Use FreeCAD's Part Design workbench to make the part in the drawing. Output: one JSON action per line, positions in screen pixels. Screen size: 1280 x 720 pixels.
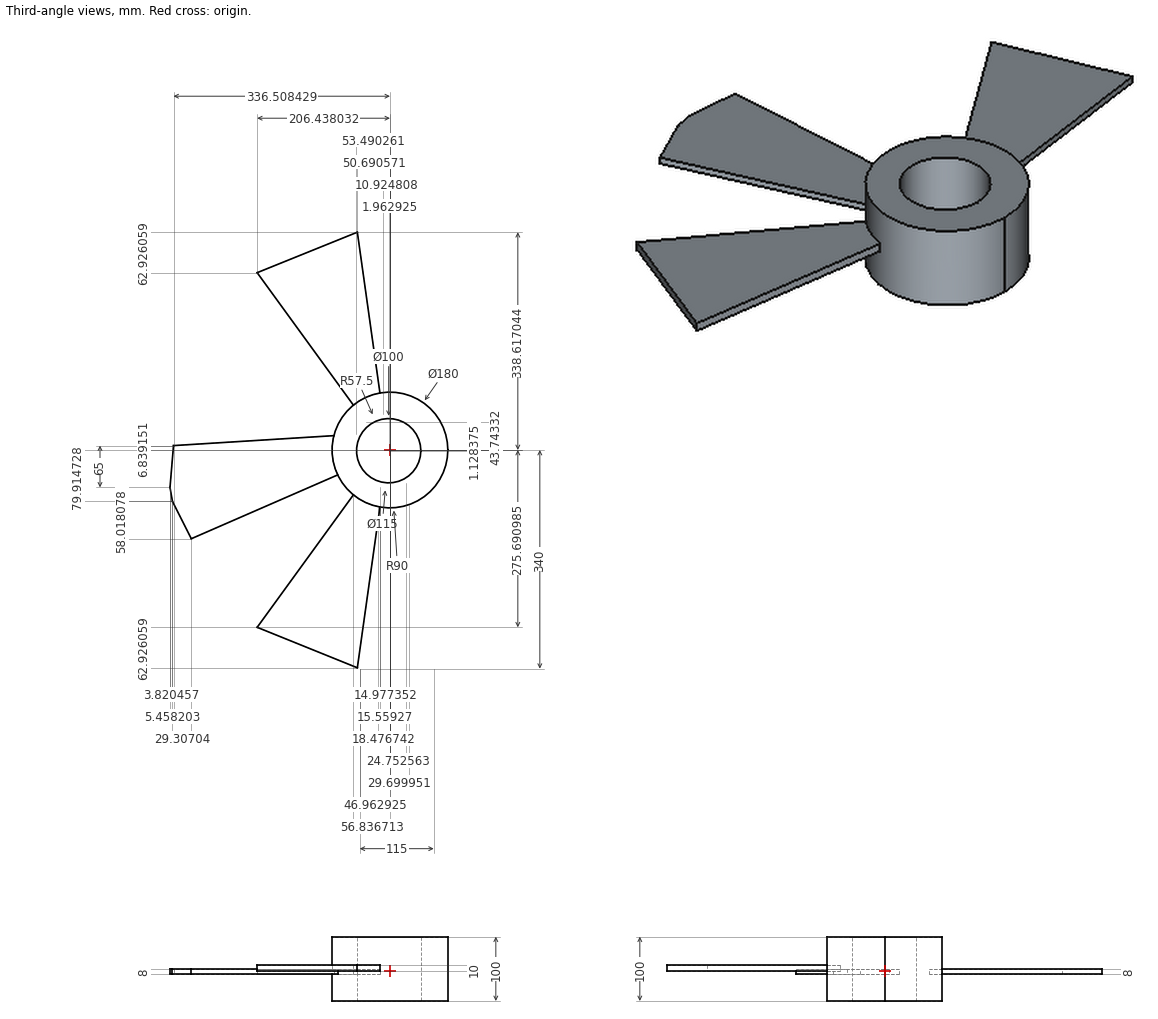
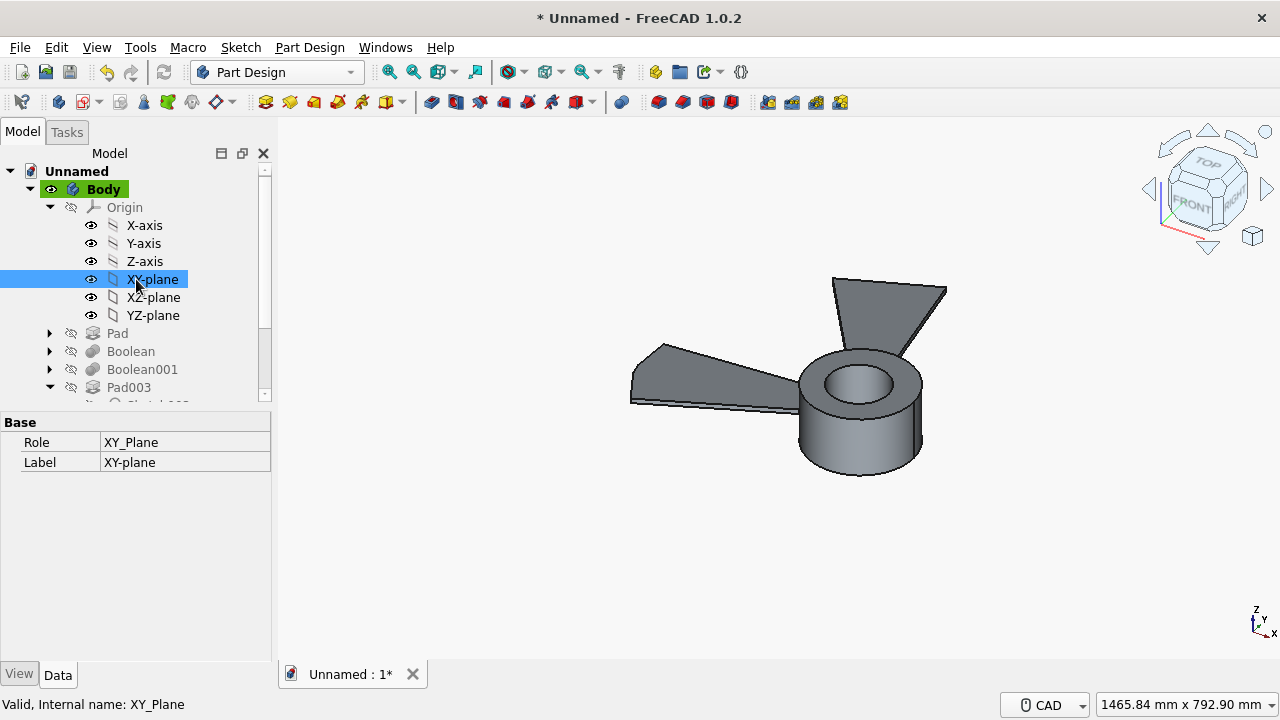
{"action": "left_click", "coordinate": [216, 102]}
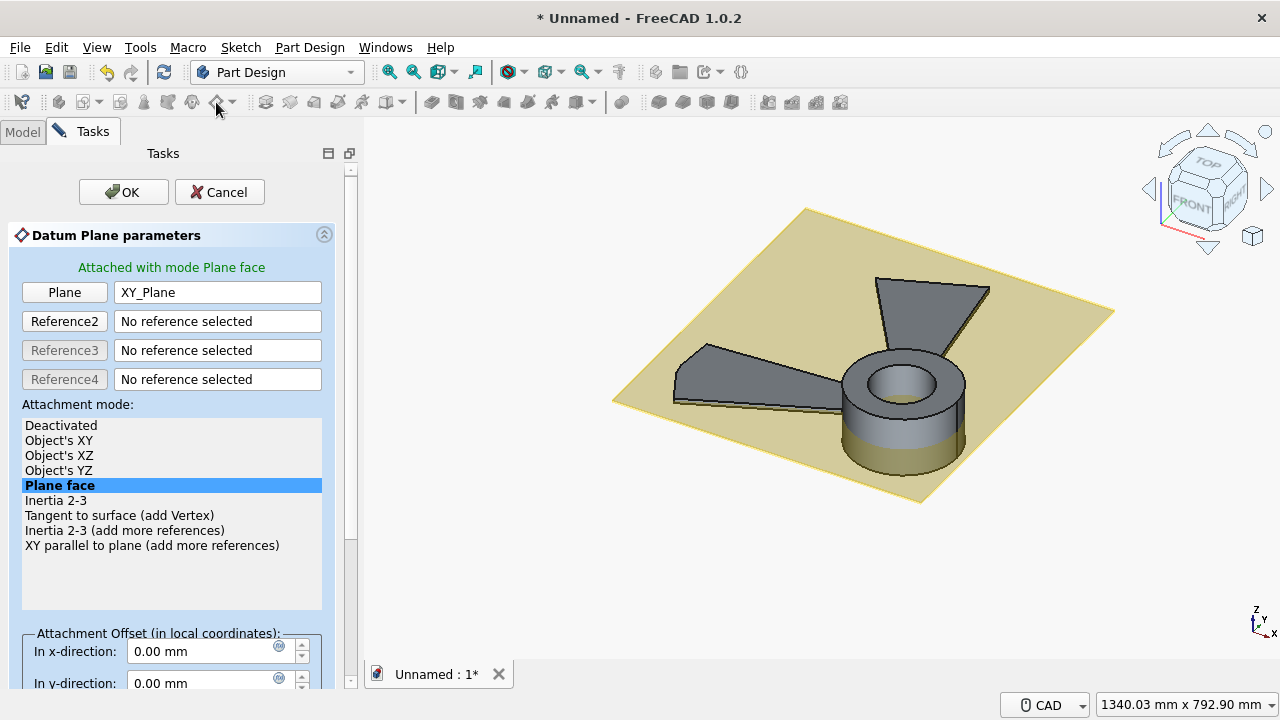
{"action": "scroll", "coordinate": [351, 426], "scroll_direction": "down", "scroll_amount": 2}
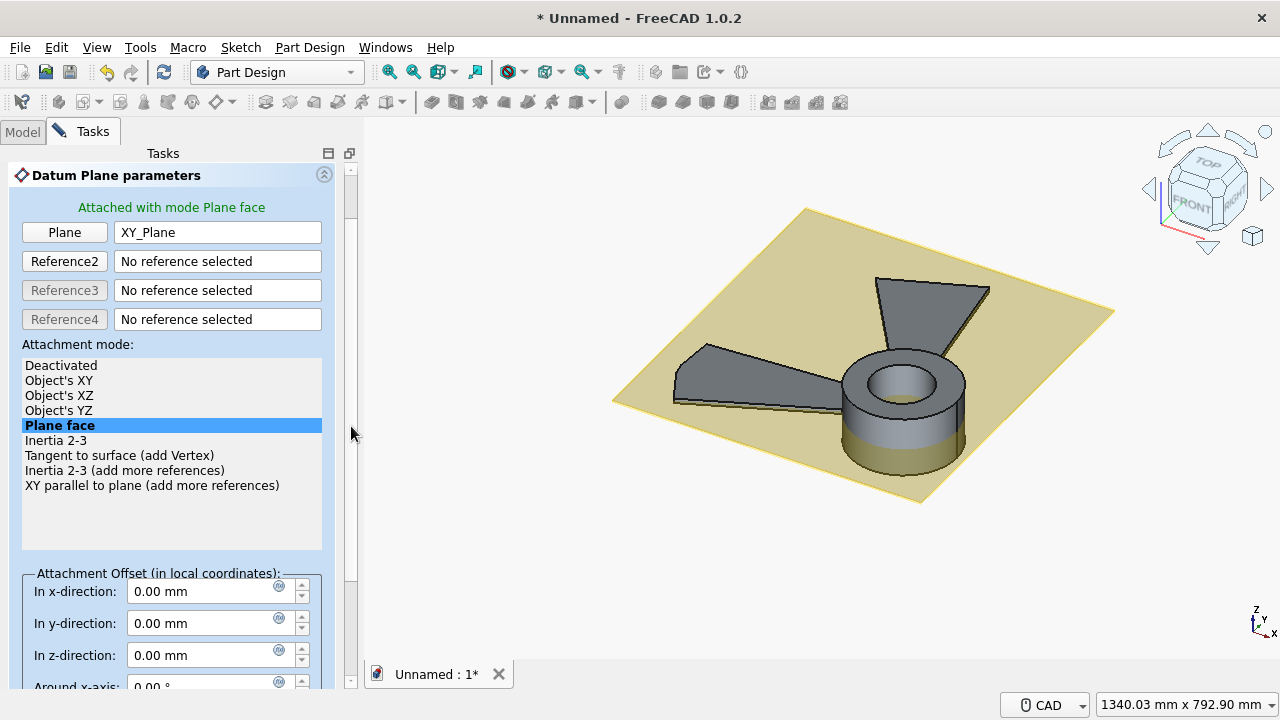
{"action": "triple_click", "coordinate": [210, 595]}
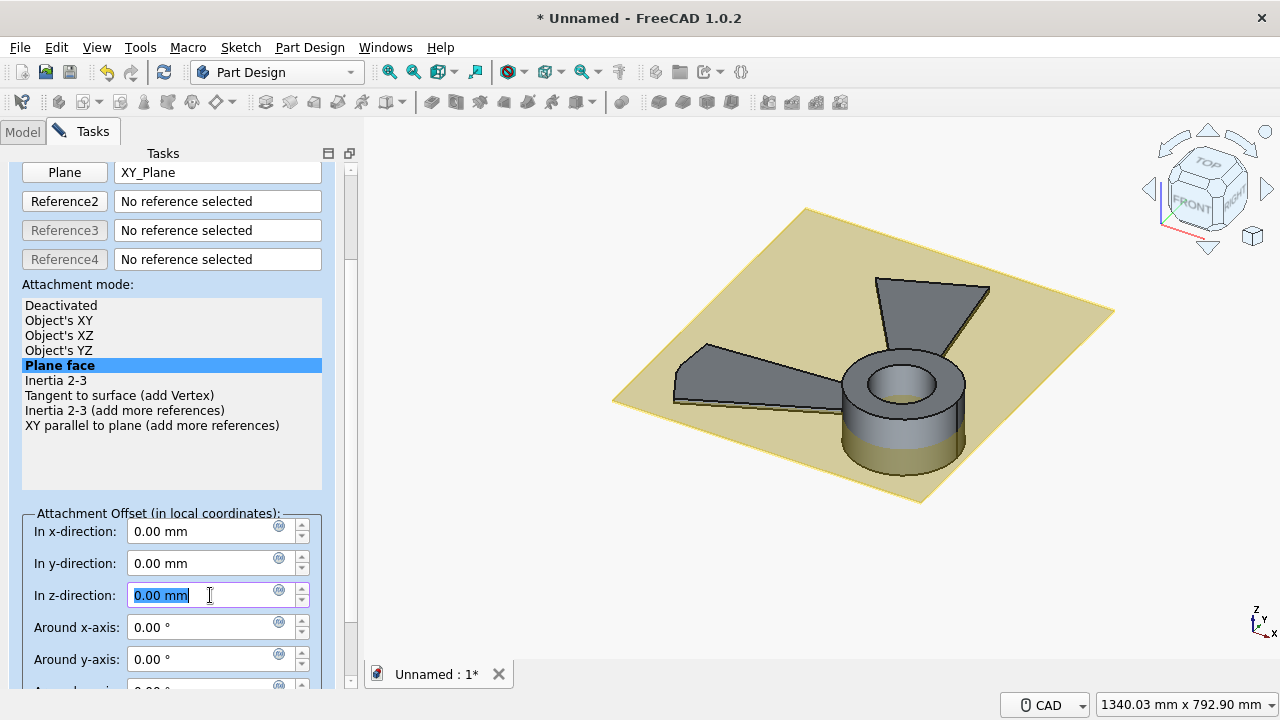
{"action": "type", "text": "10"}
{"action": "key", "text": "Tab"}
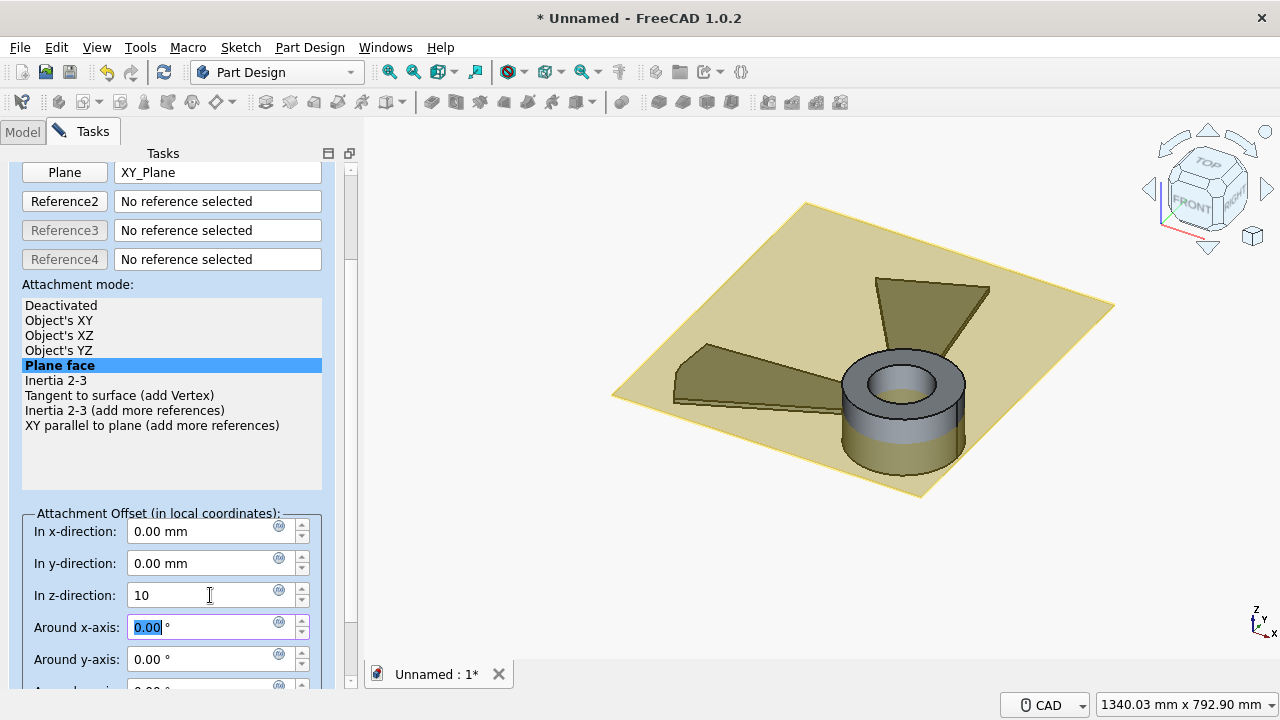
{"action": "scroll", "coordinate": [351, 426], "scroll_direction": "up", "scroll_amount": 3}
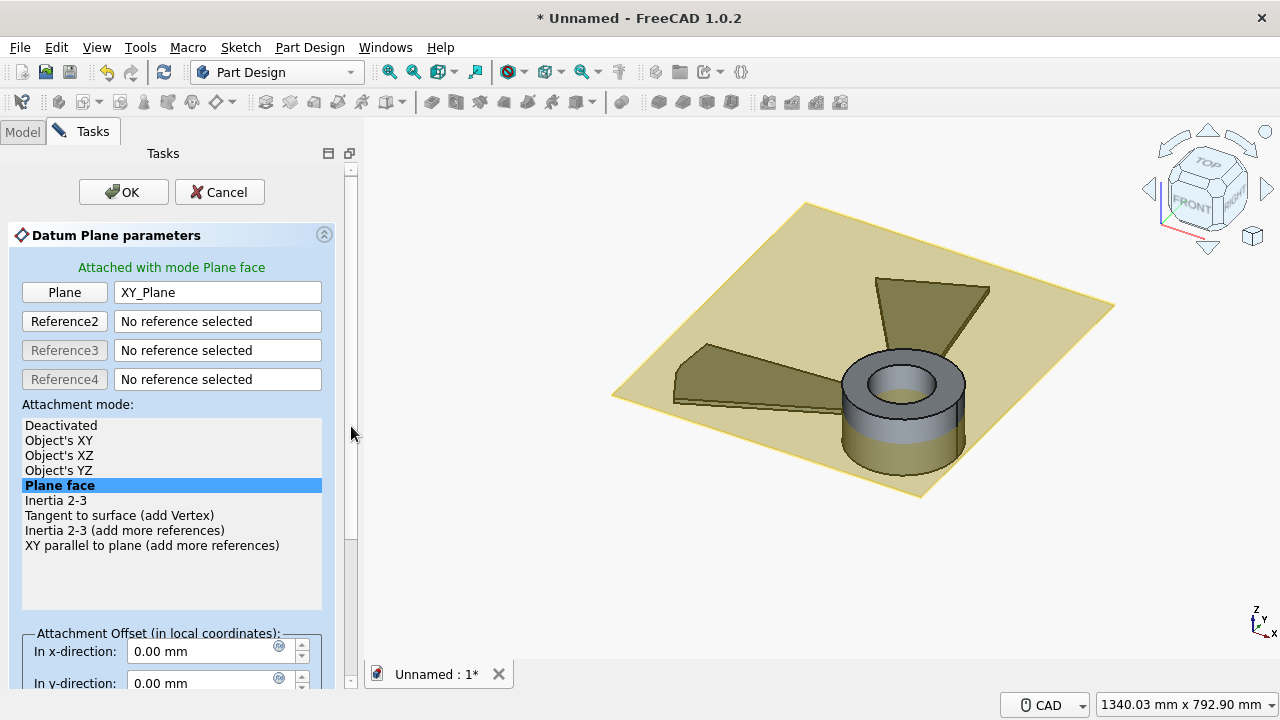
{"action": "left_click", "coordinate": [124, 192]}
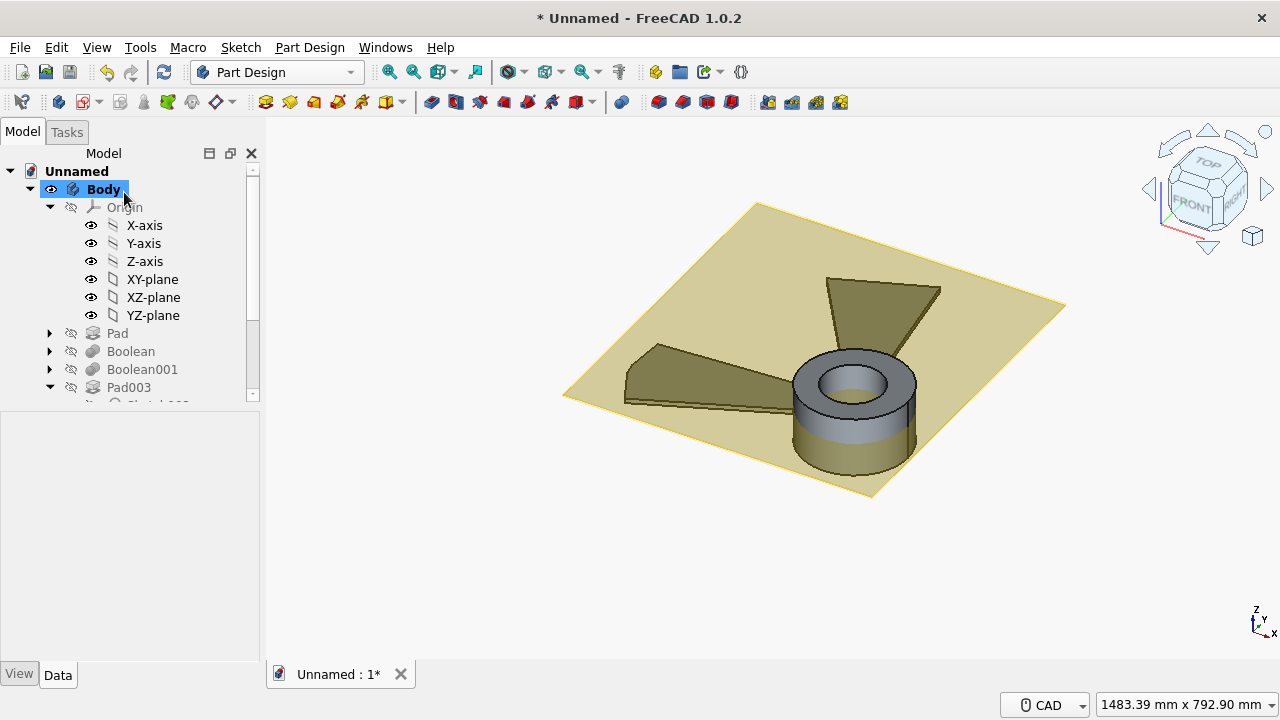
{"action": "scroll", "coordinate": [100, 275], "scroll_direction": "down", "scroll_amount": 3}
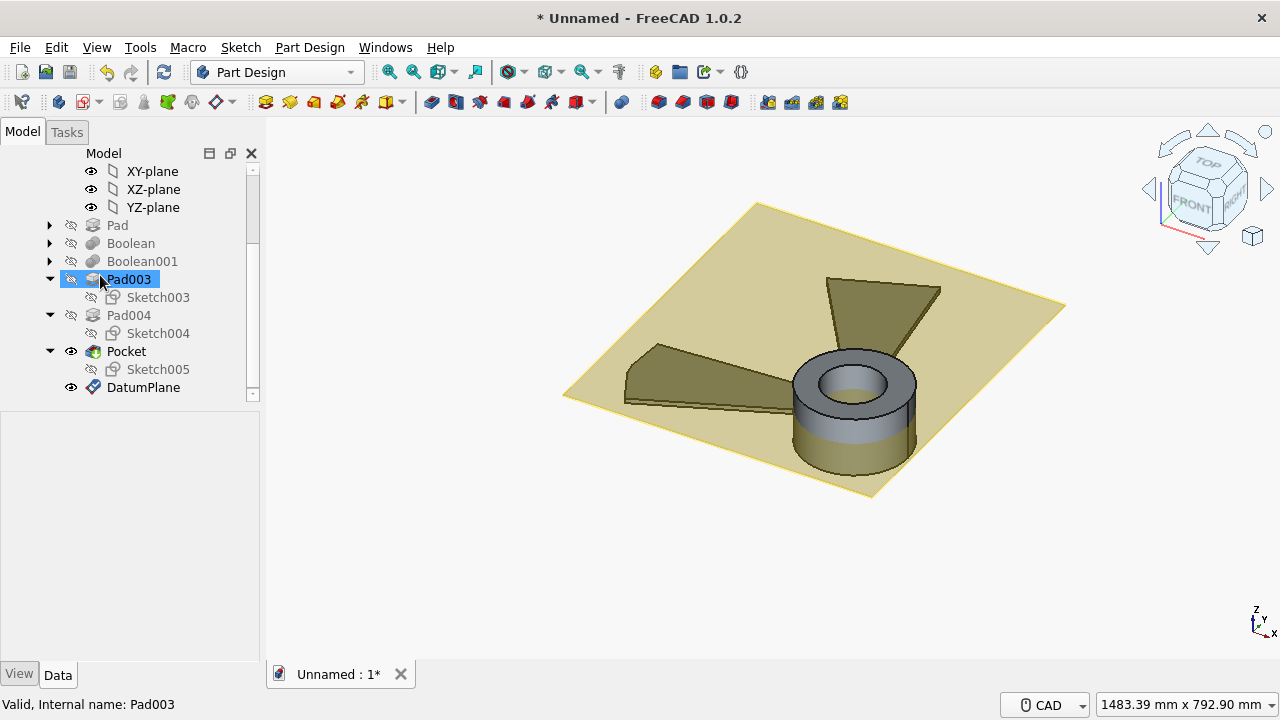
{"action": "left_click", "coordinate": [116, 387]}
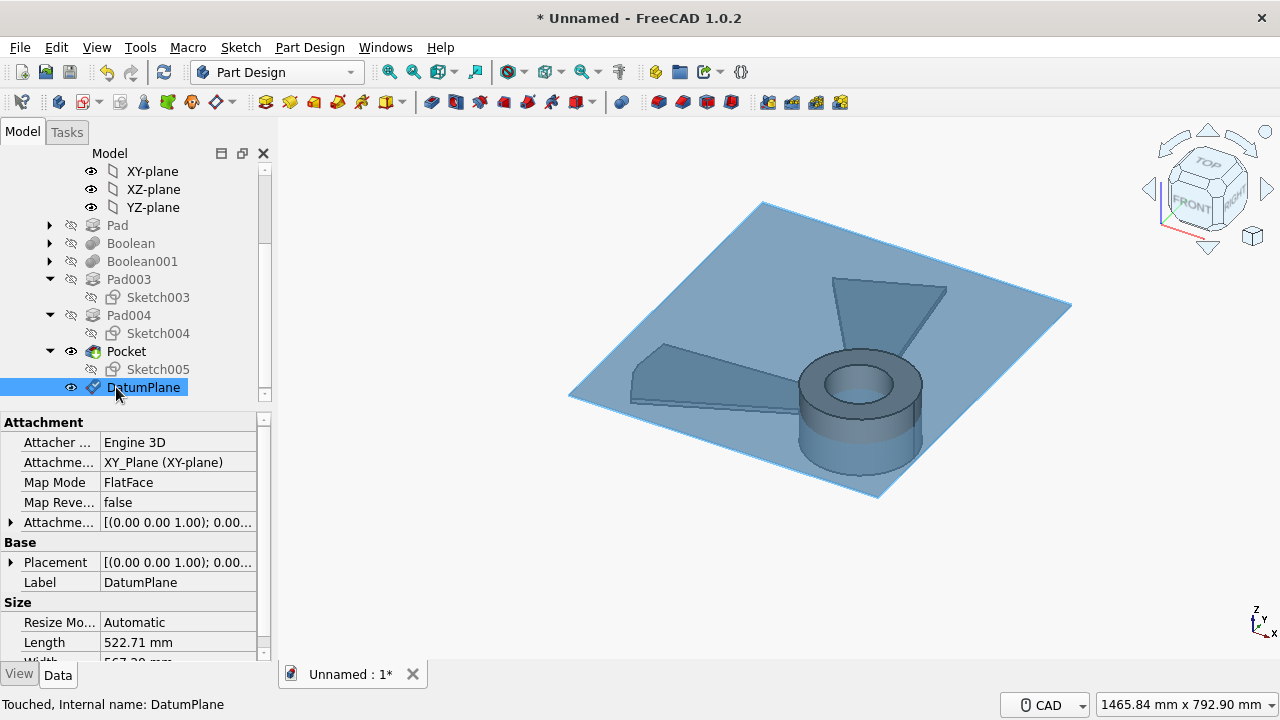
{"action": "left_click", "coordinate": [84, 102]}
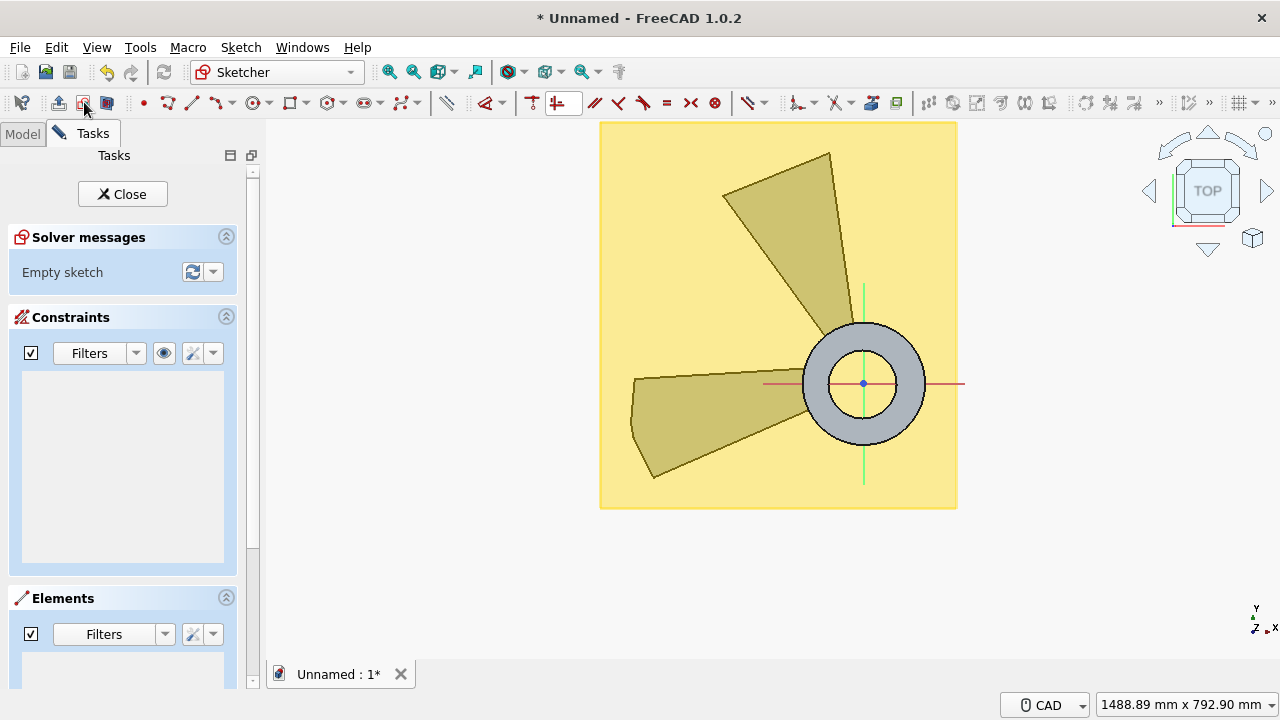
{"action": "left_click", "coordinate": [108, 104]}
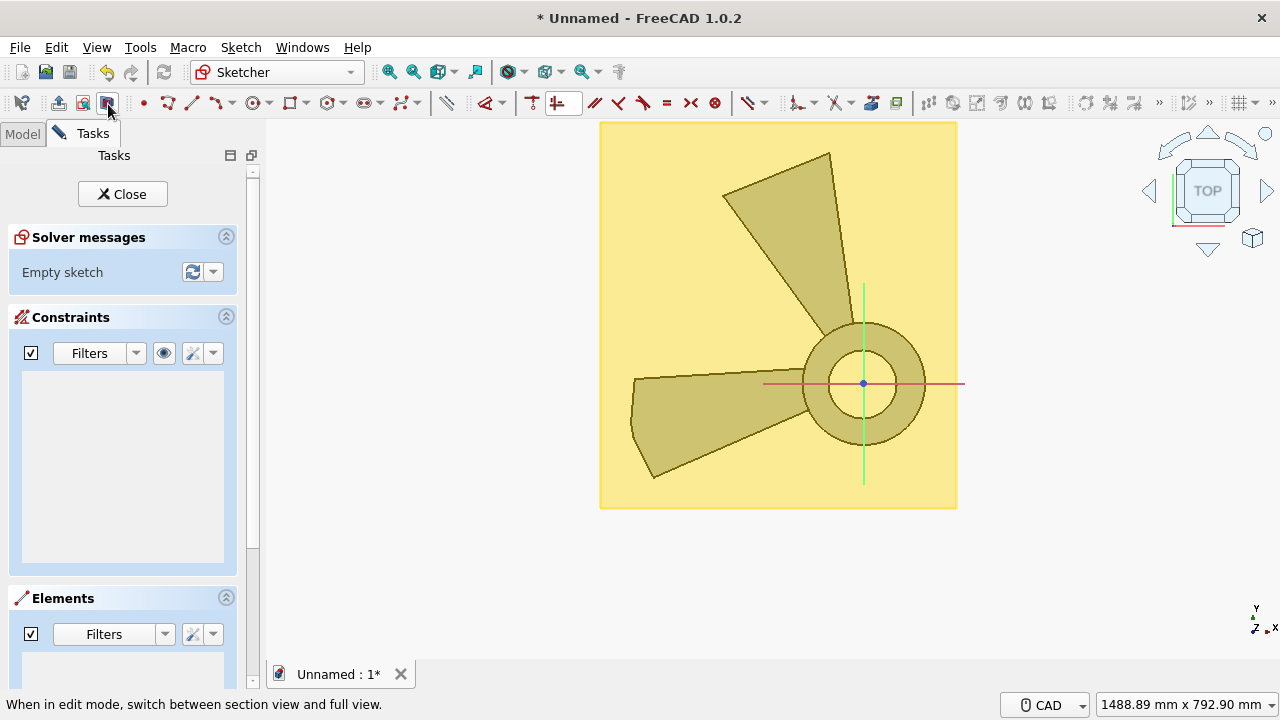
{"action": "scroll", "coordinate": [302, 147], "scroll_direction": "down", "scroll_amount": 1}